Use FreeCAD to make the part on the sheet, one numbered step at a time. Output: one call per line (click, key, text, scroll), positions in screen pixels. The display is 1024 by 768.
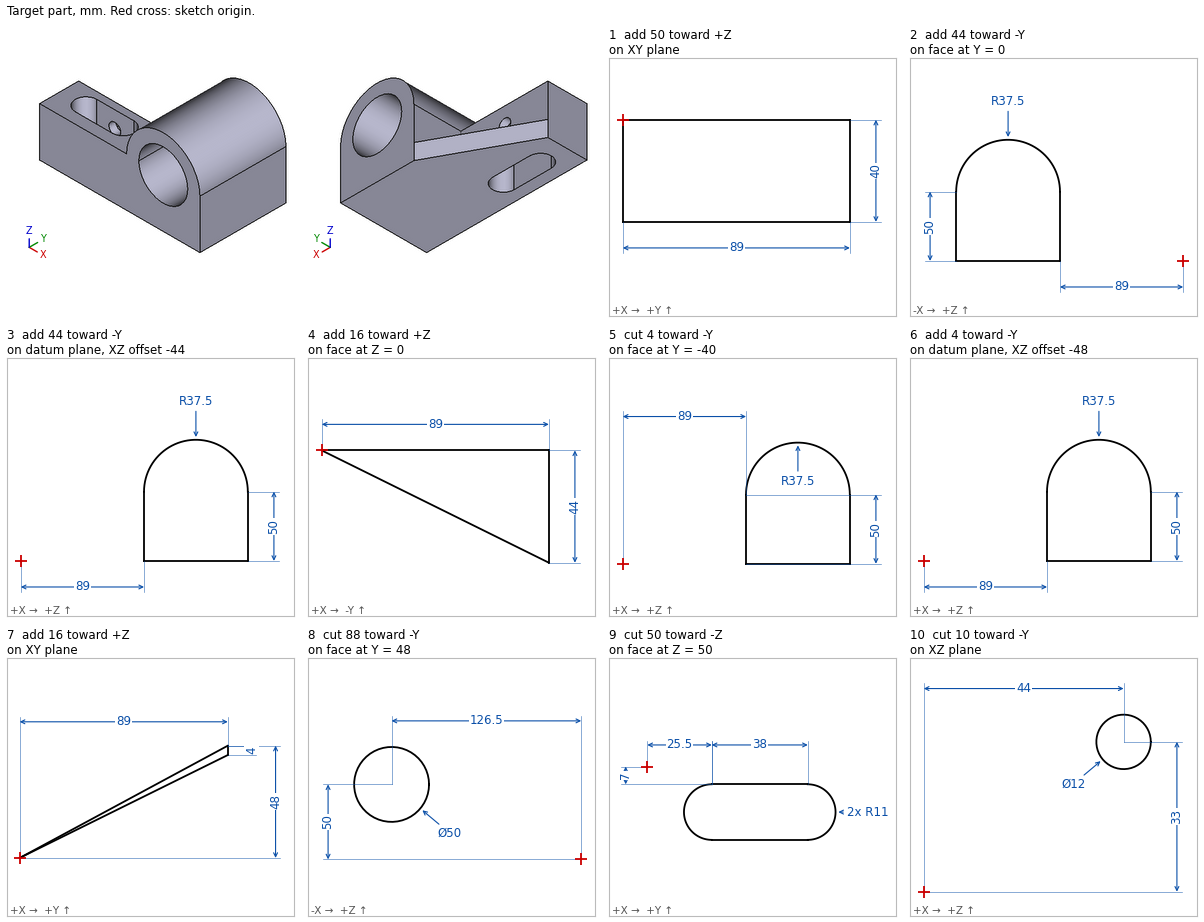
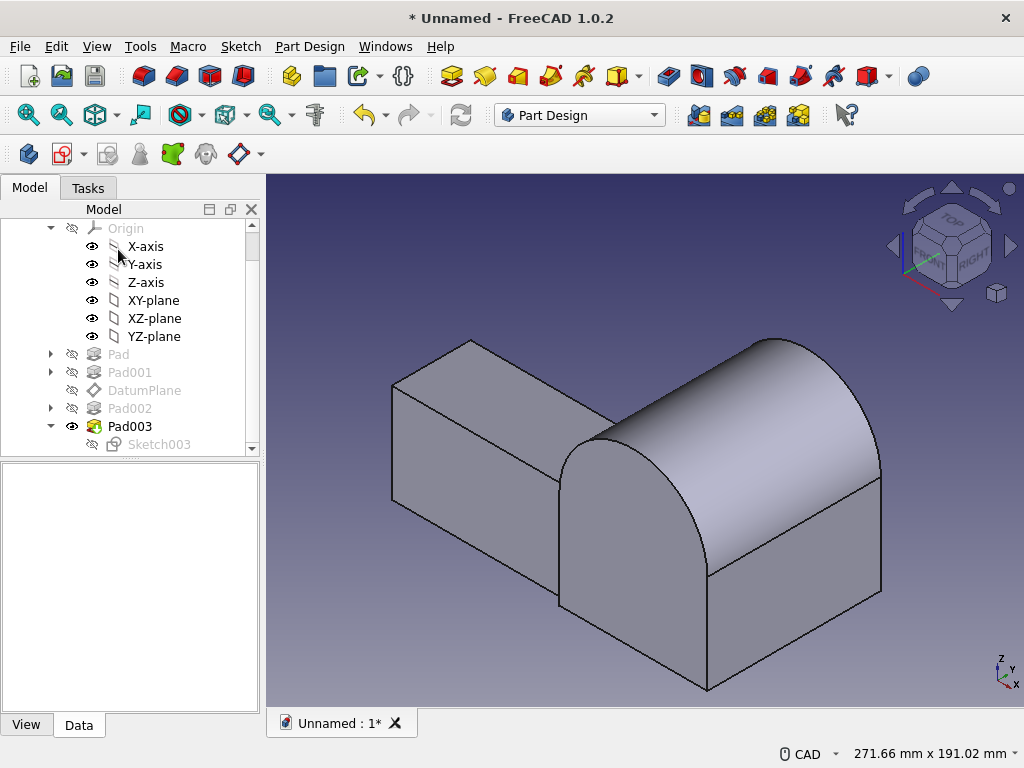
click(505, 507)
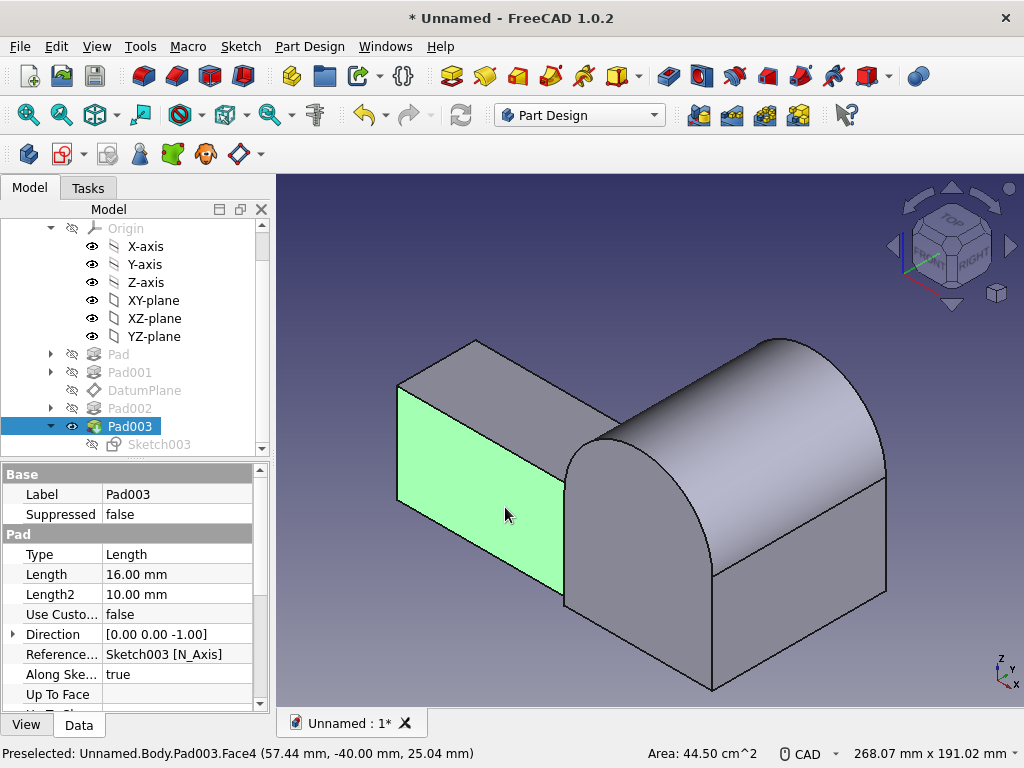
click(62, 154)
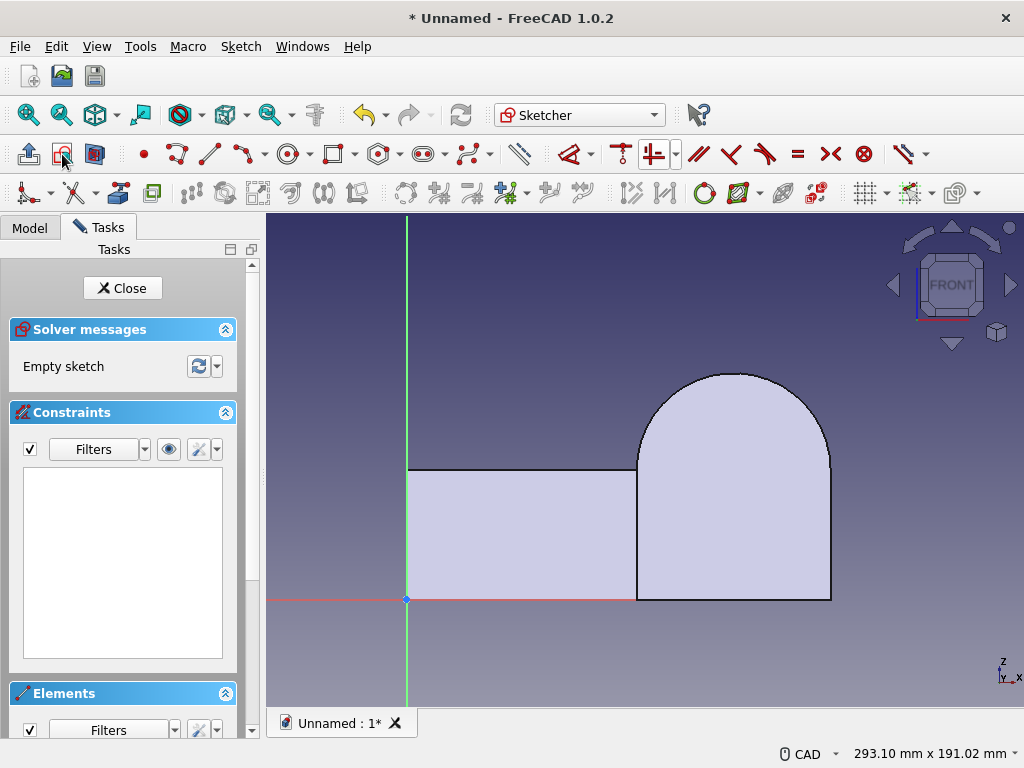
key(q)
key(s)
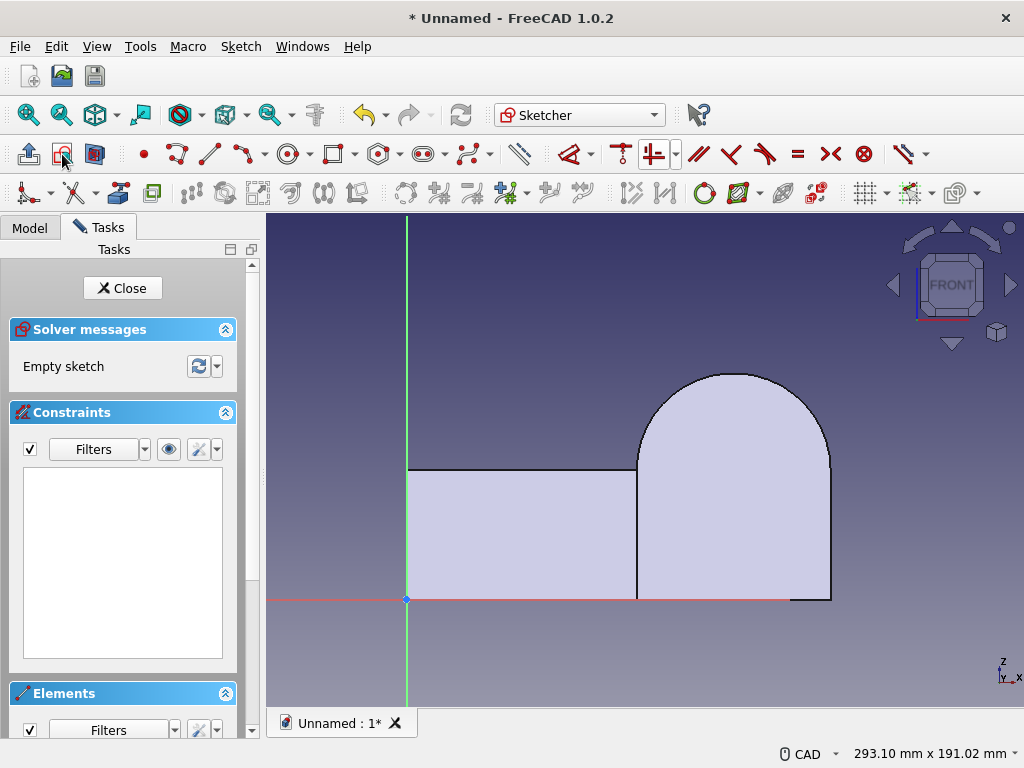
click(177, 154)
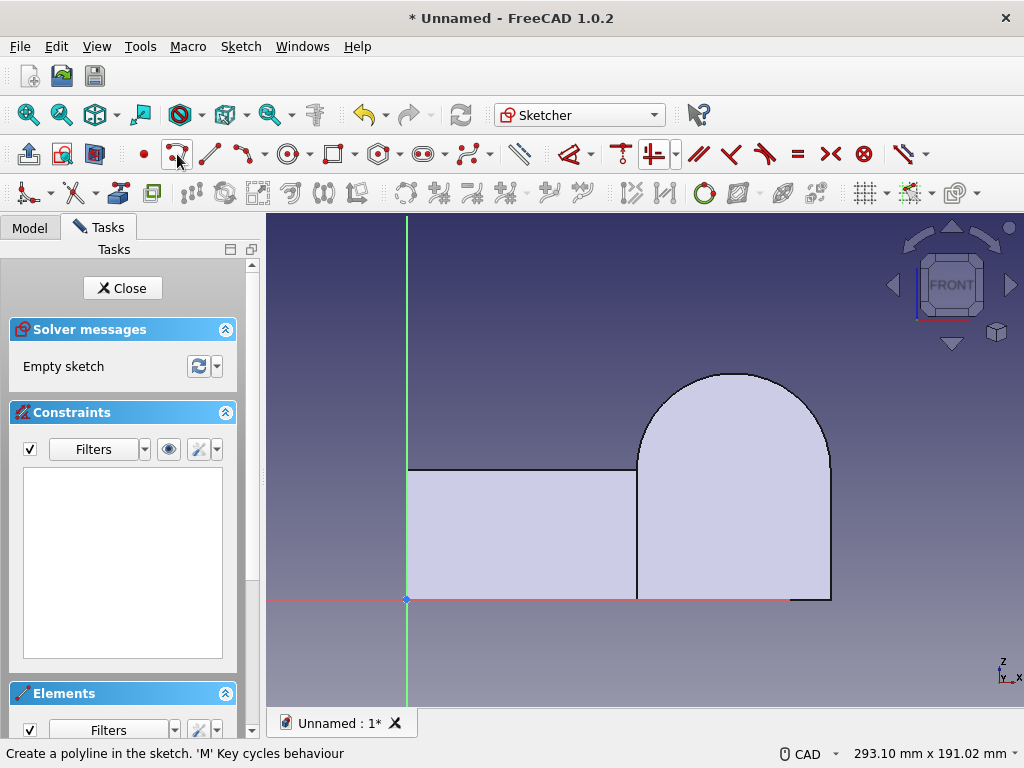
click(637, 470)
click(637, 600)
click(831, 591)
click(831, 470)
right_click(831, 470)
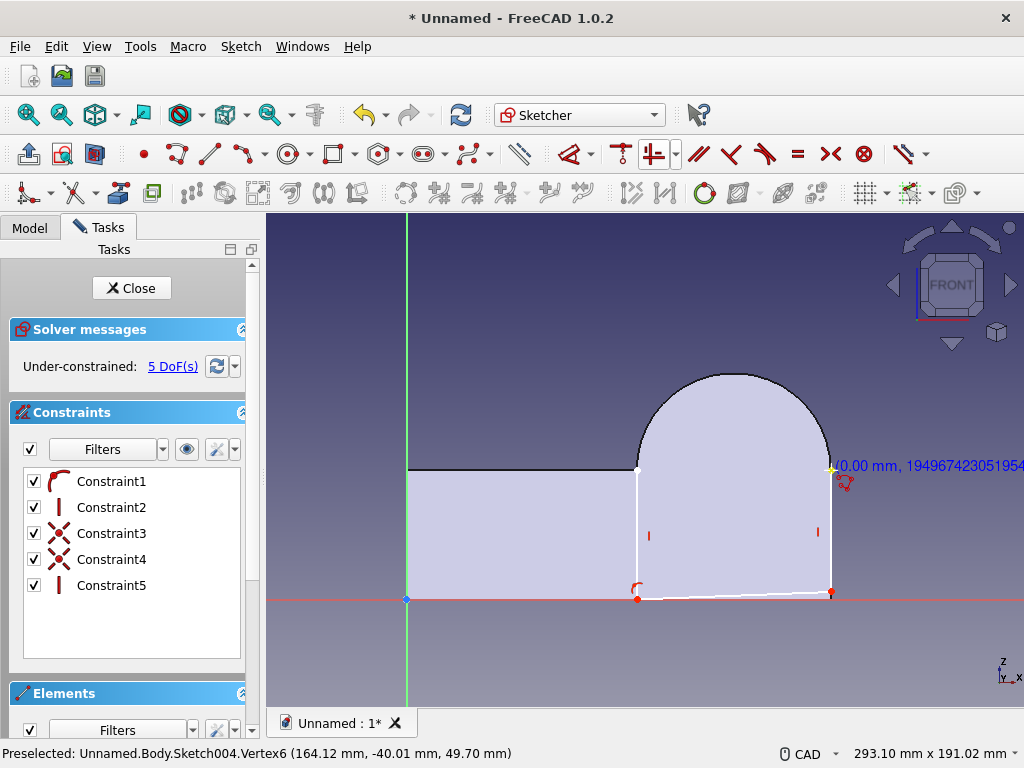
click(242, 154)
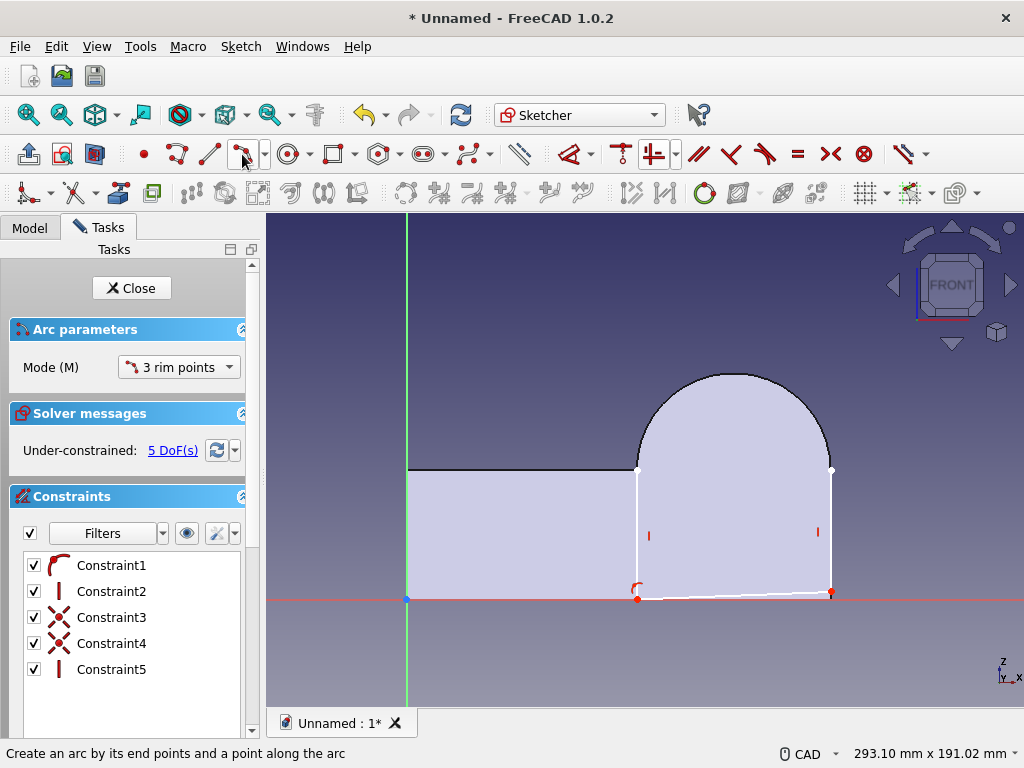
click(831, 471)
click(637, 471)
click(734, 373)
key(Escape)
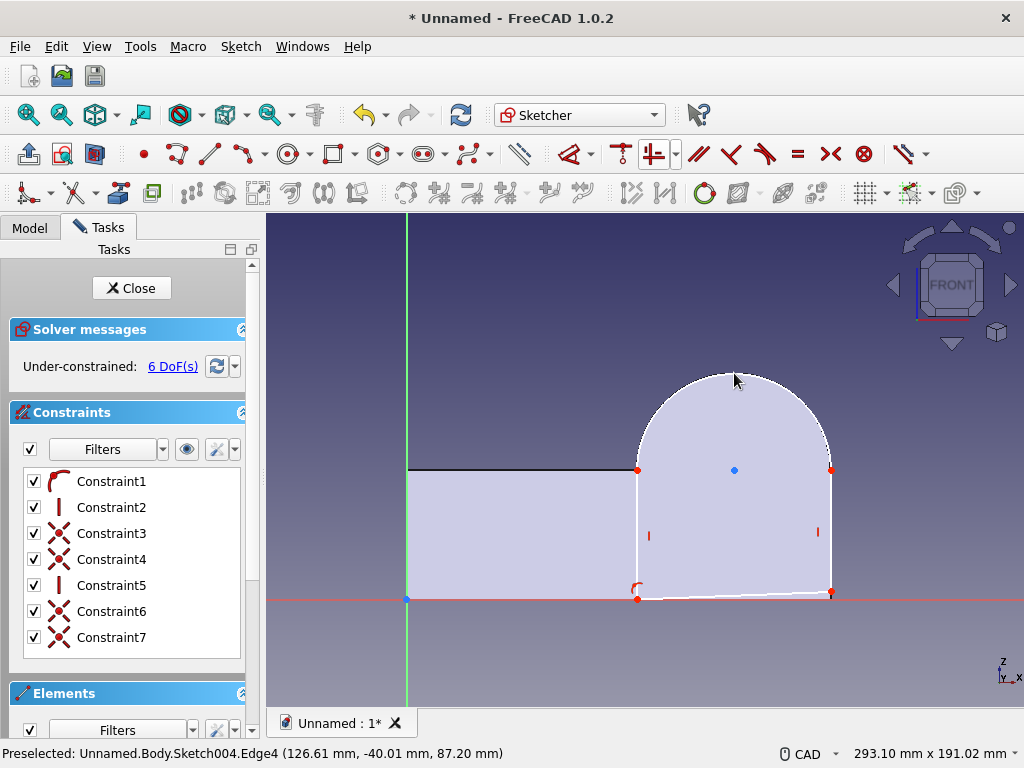
click(637, 510)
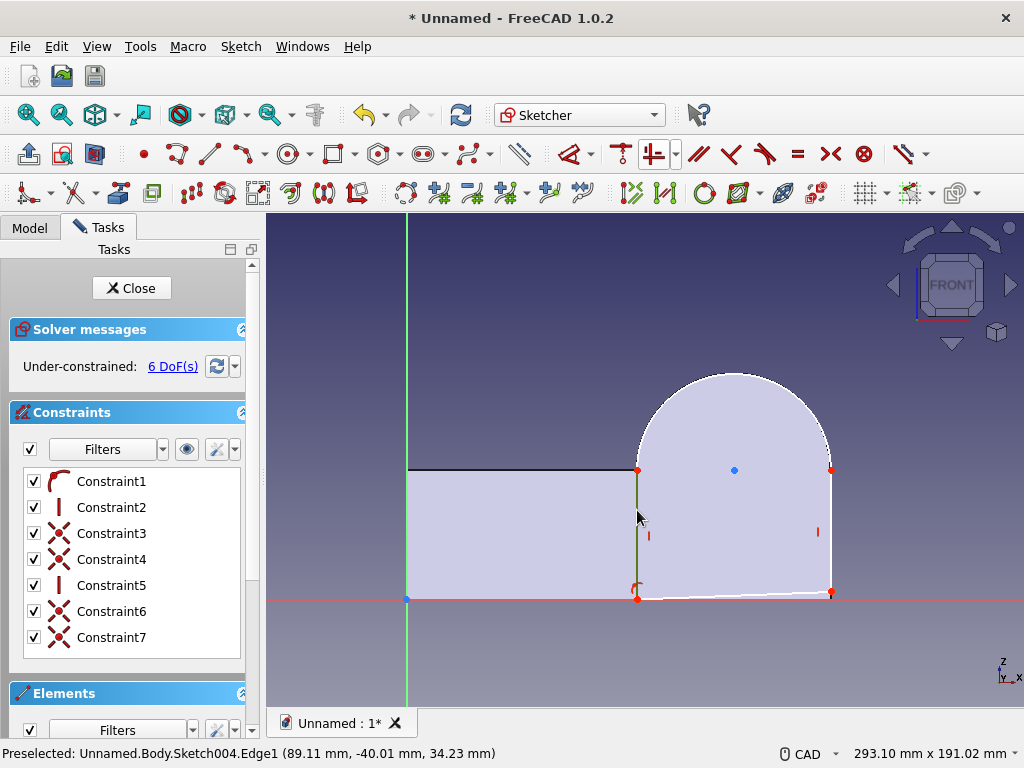
click(791, 393)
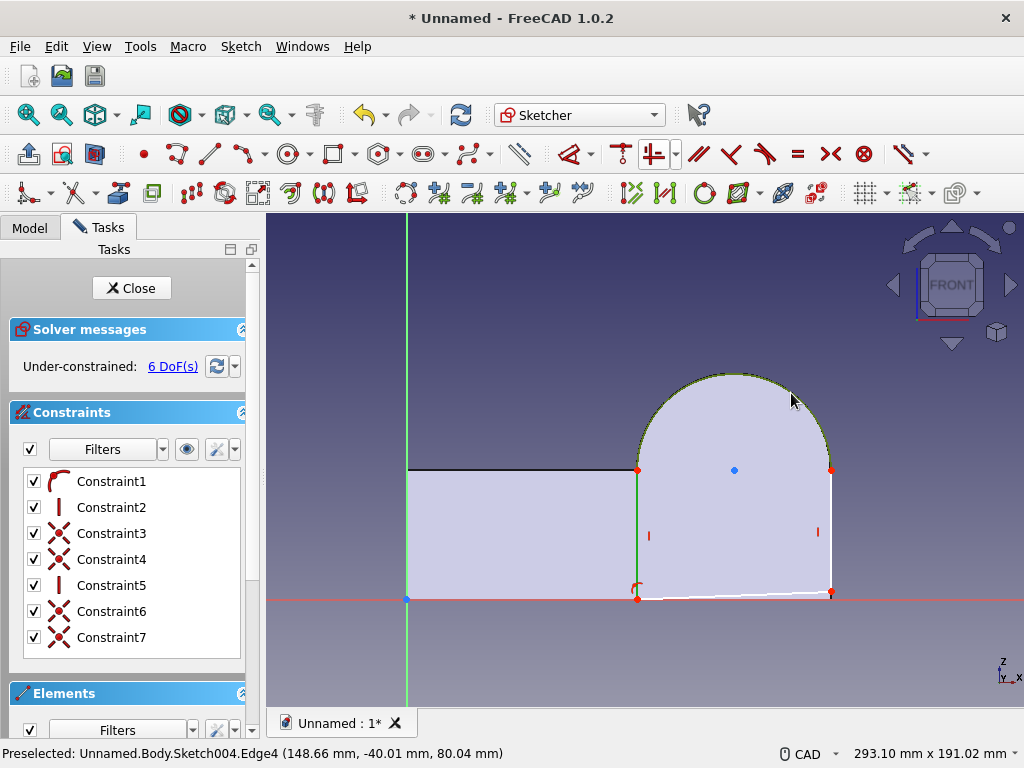
click(765, 154)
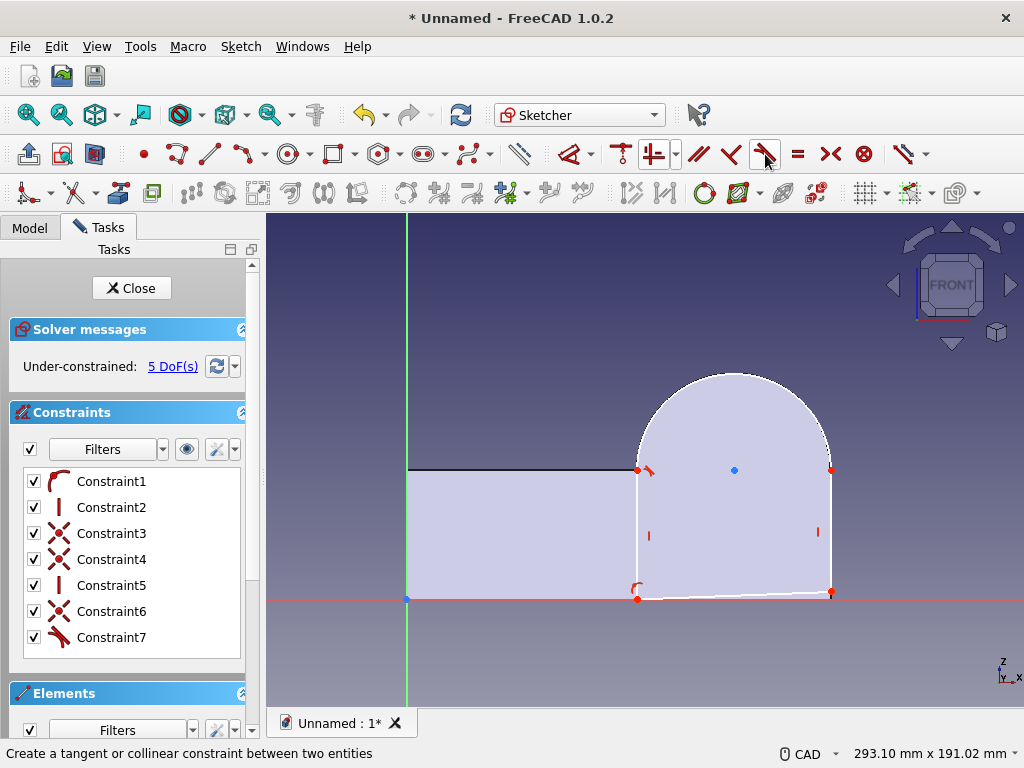
click(831, 556)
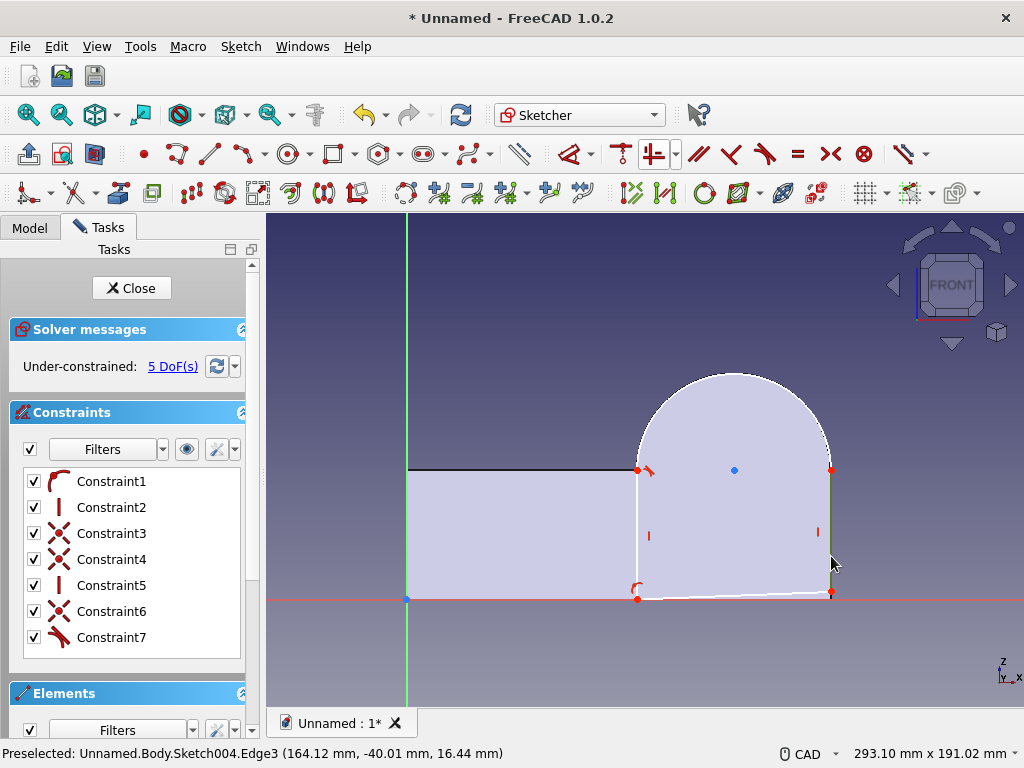
click(791, 393)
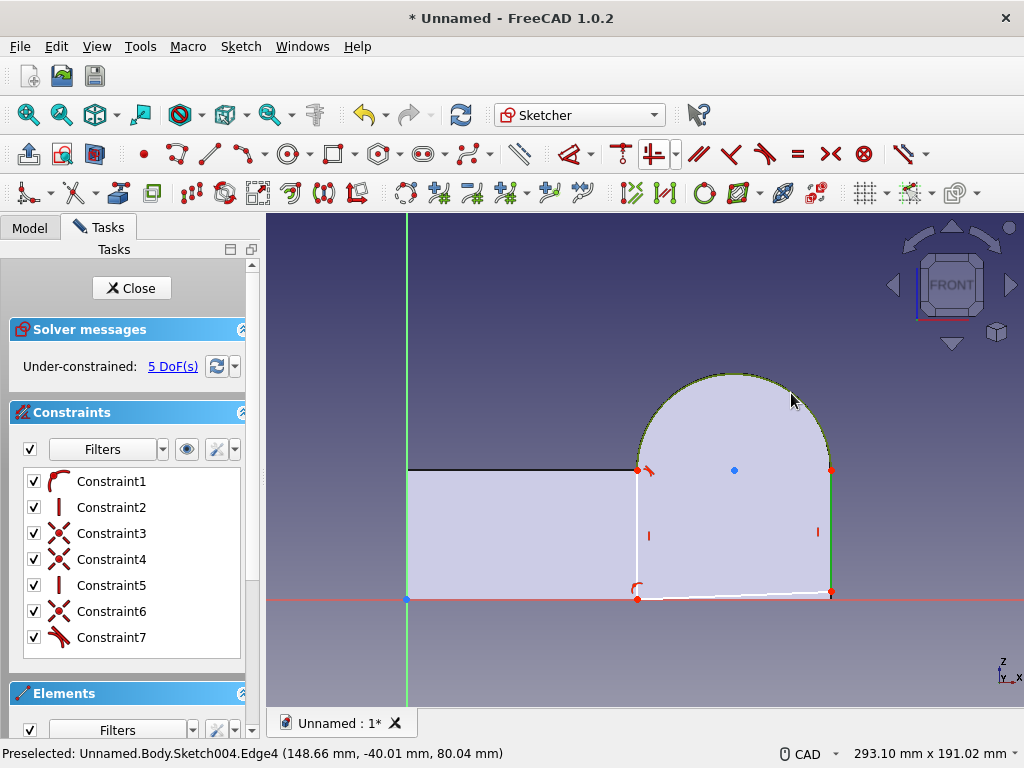
click(765, 154)